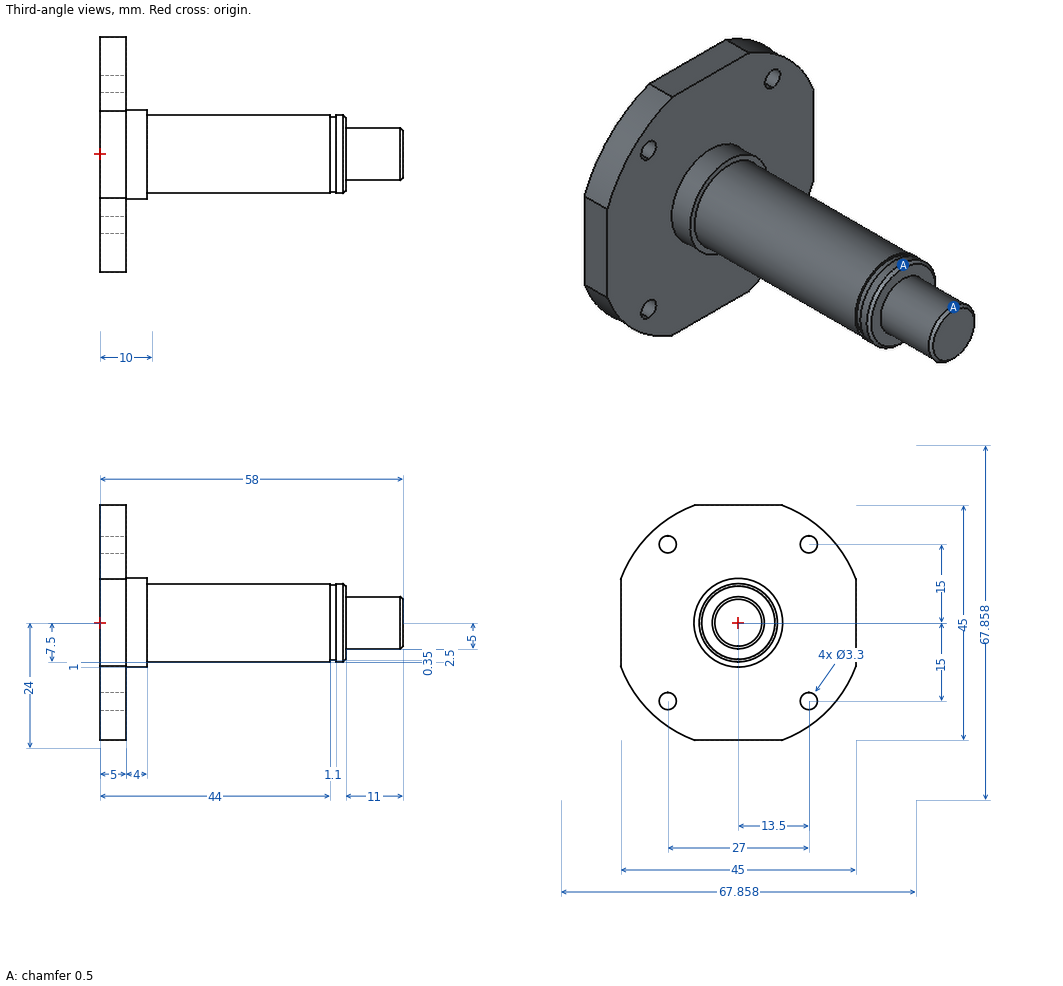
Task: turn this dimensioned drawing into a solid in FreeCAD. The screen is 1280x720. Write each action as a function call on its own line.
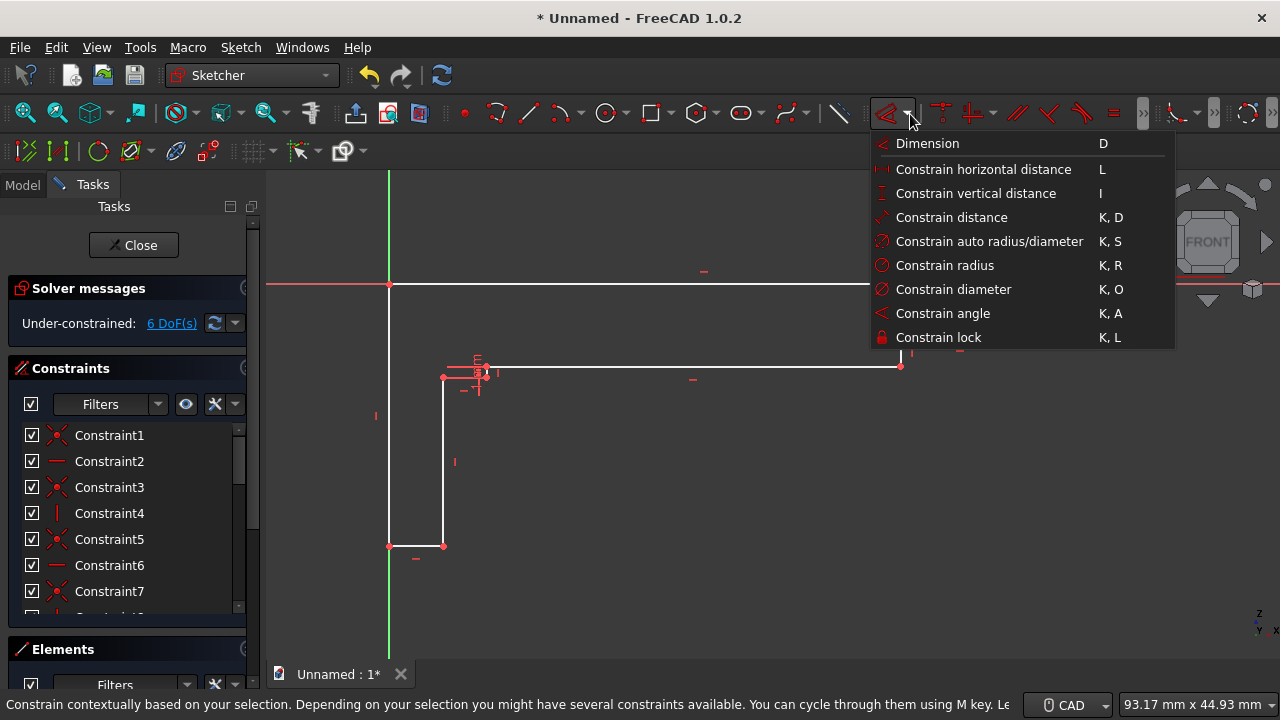
click(1023, 169)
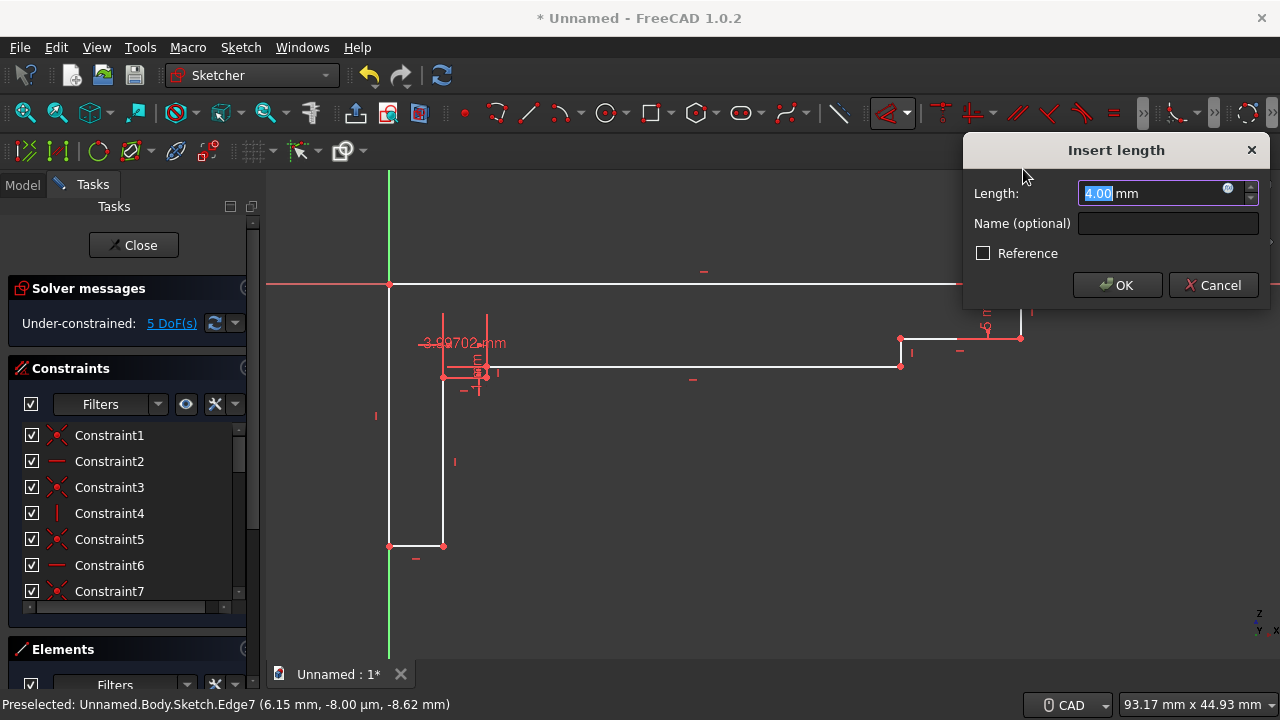
text(4)
key(Return)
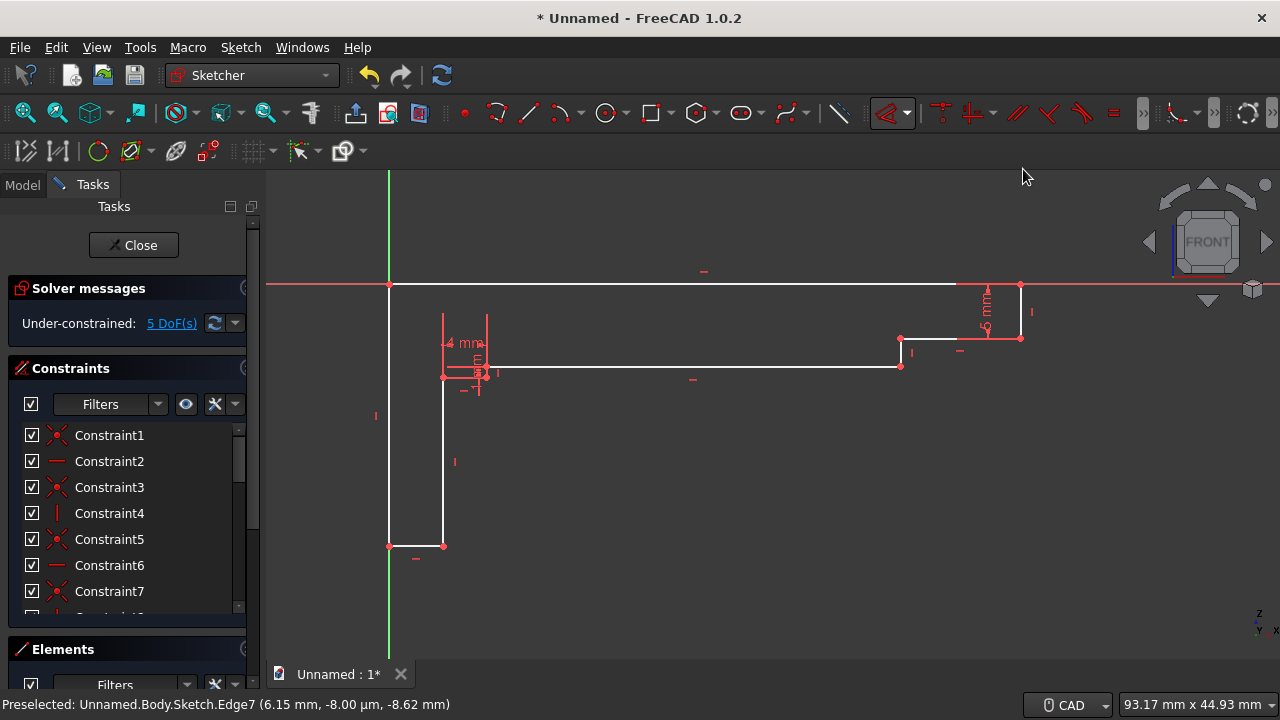
click(427, 546)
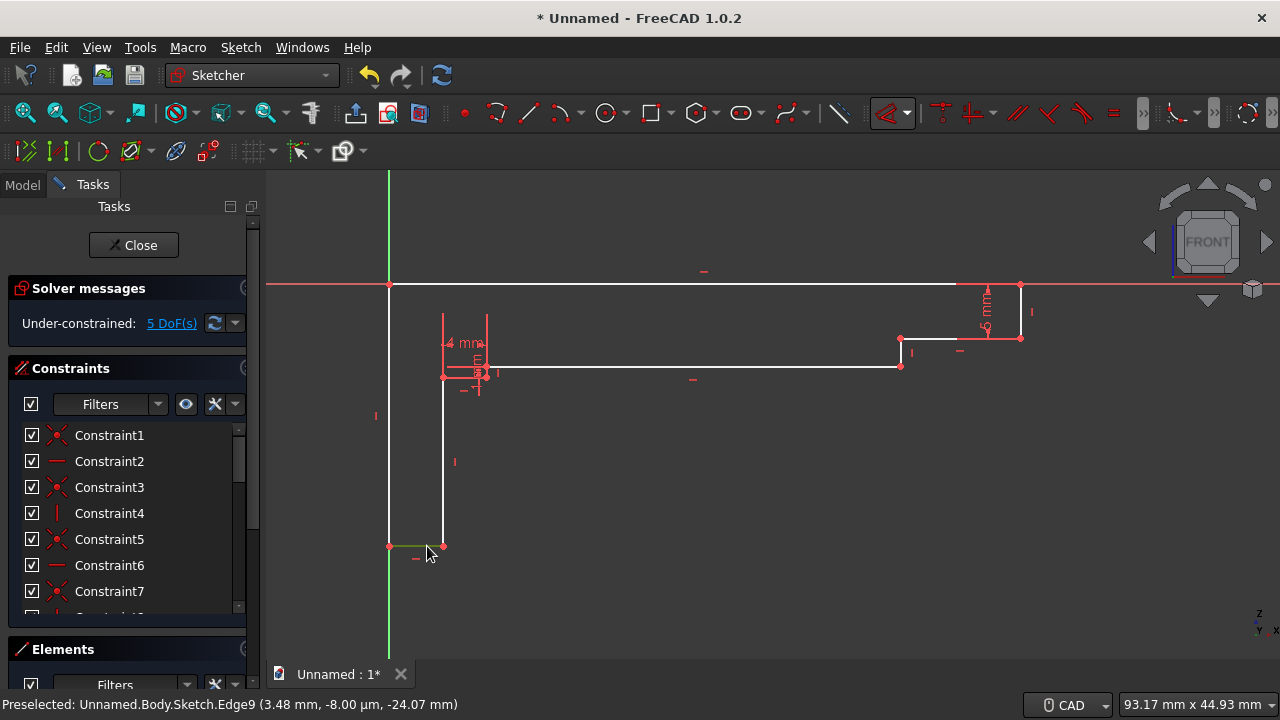
key(l)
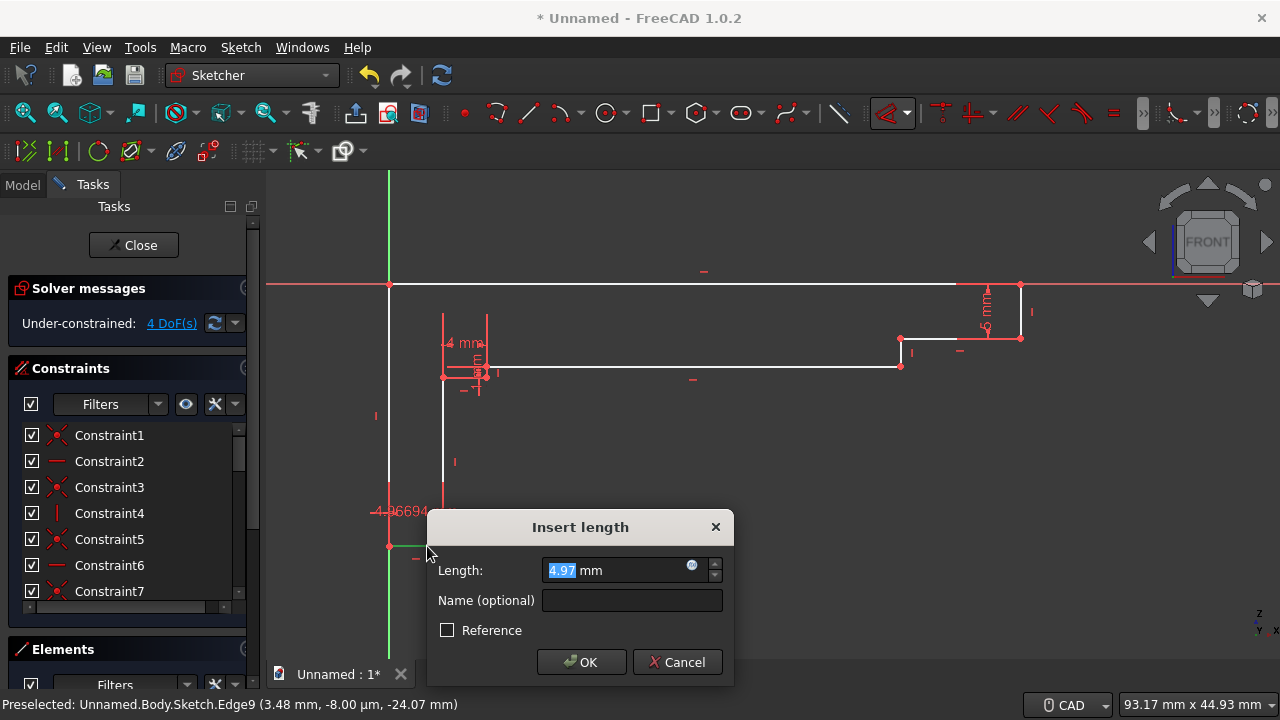
text(5)
key(Return)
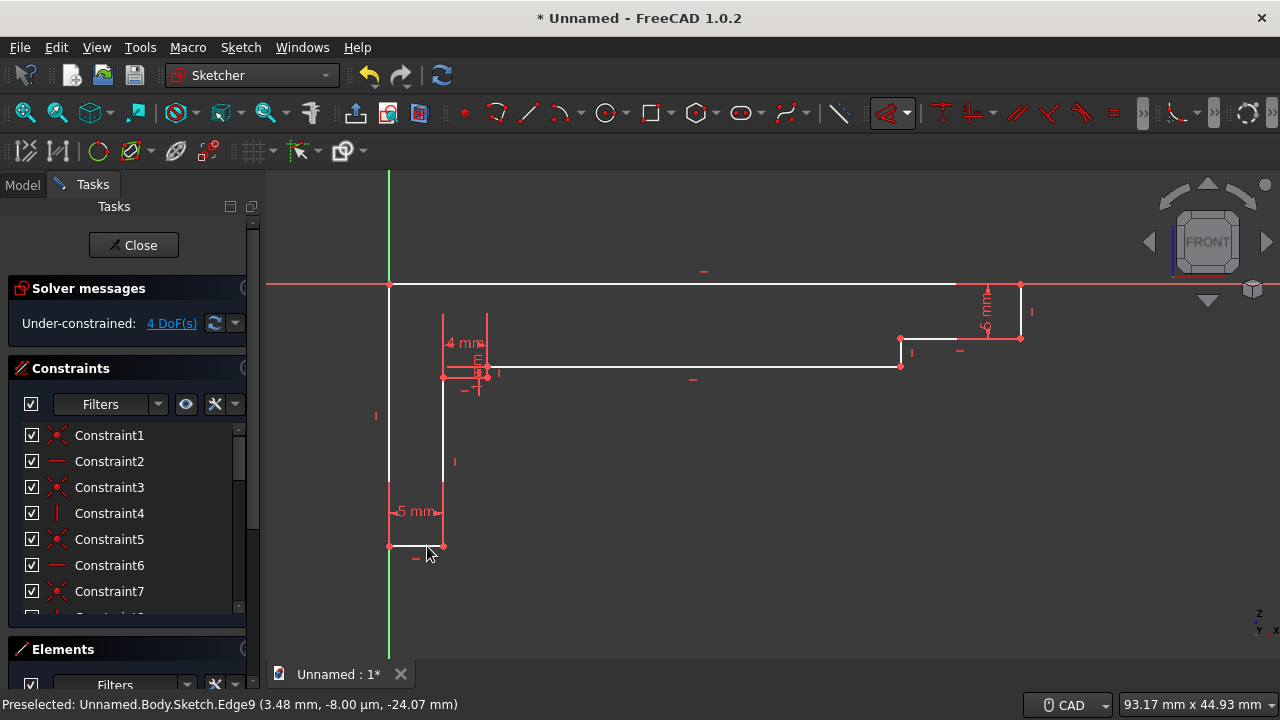
click(579, 284)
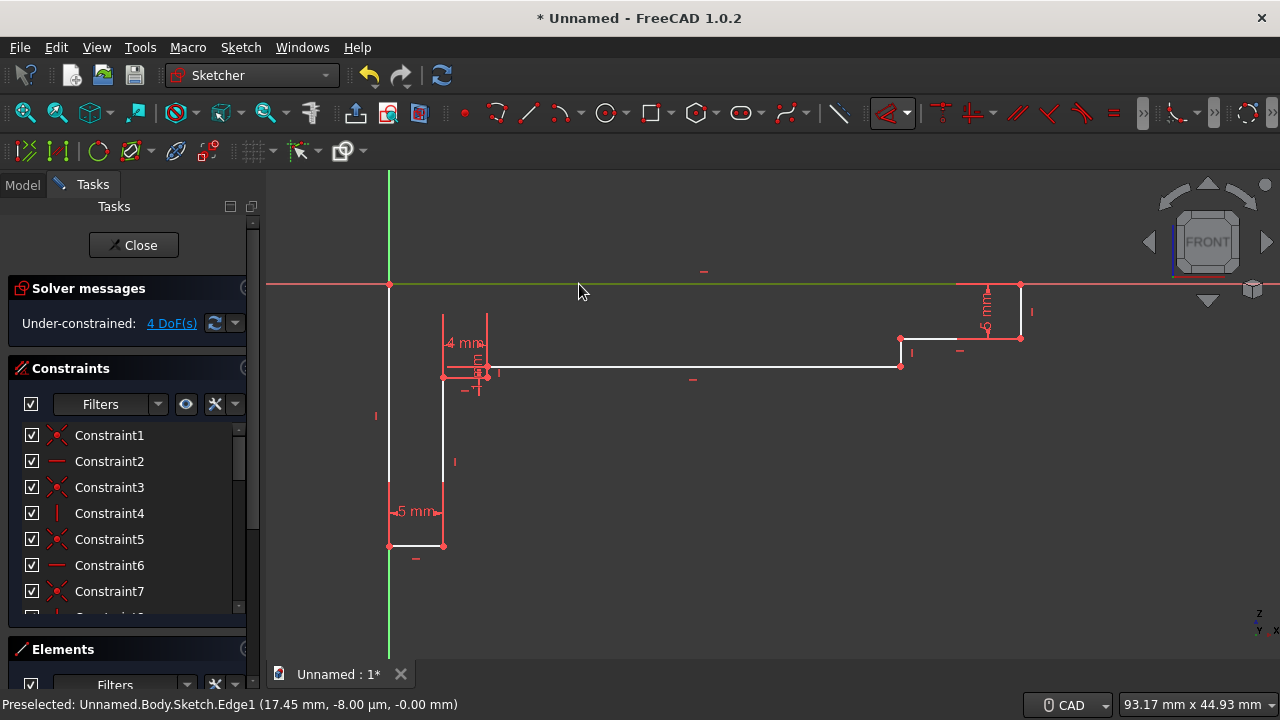
key(l)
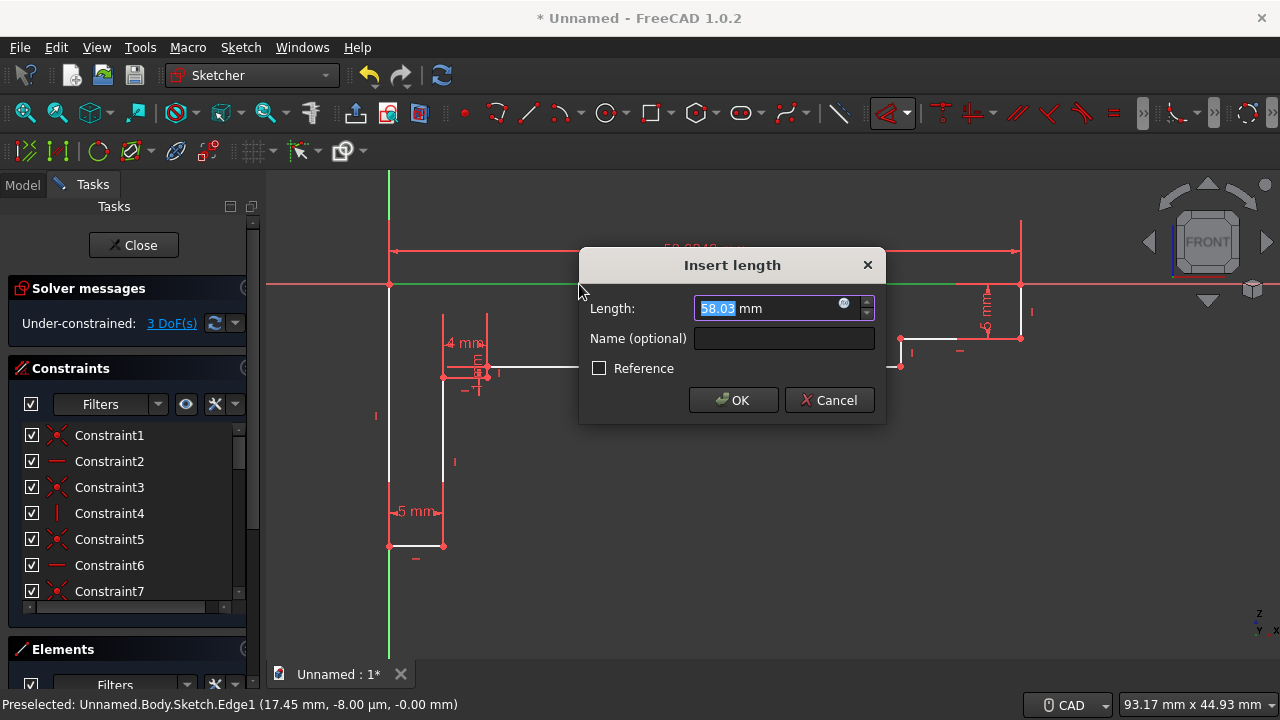
text(58)
key(Return)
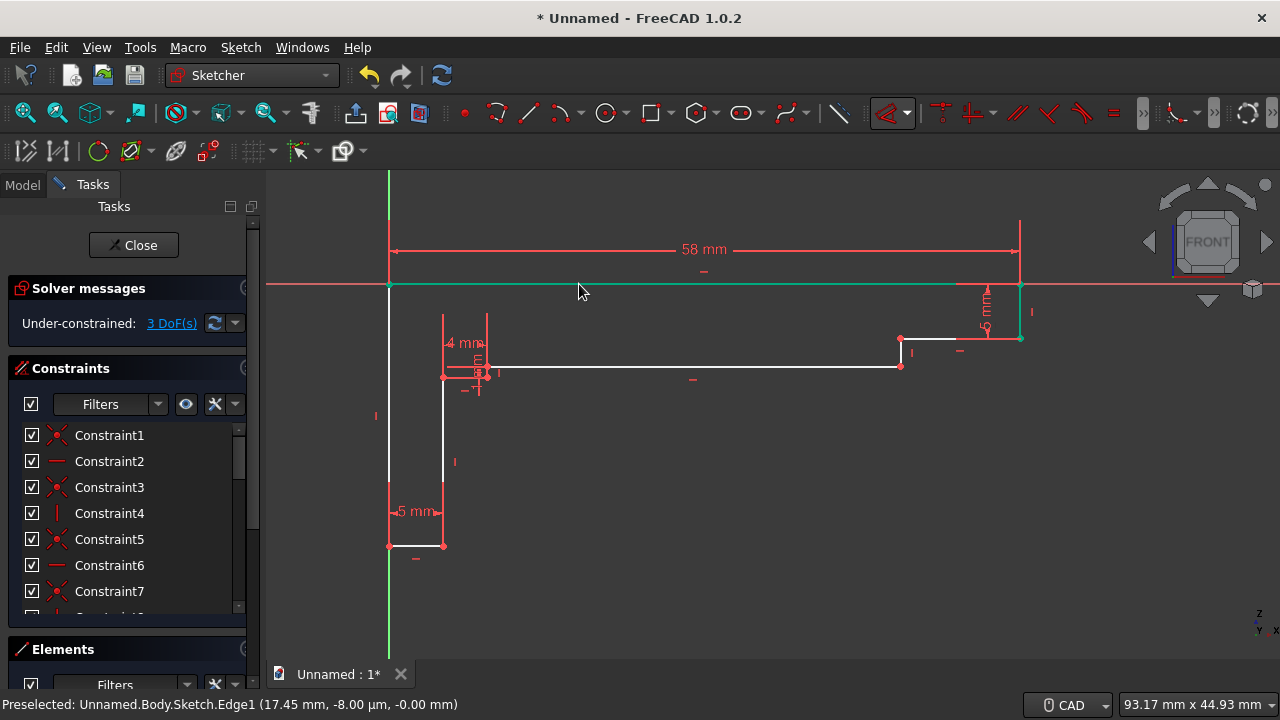
click(984, 339)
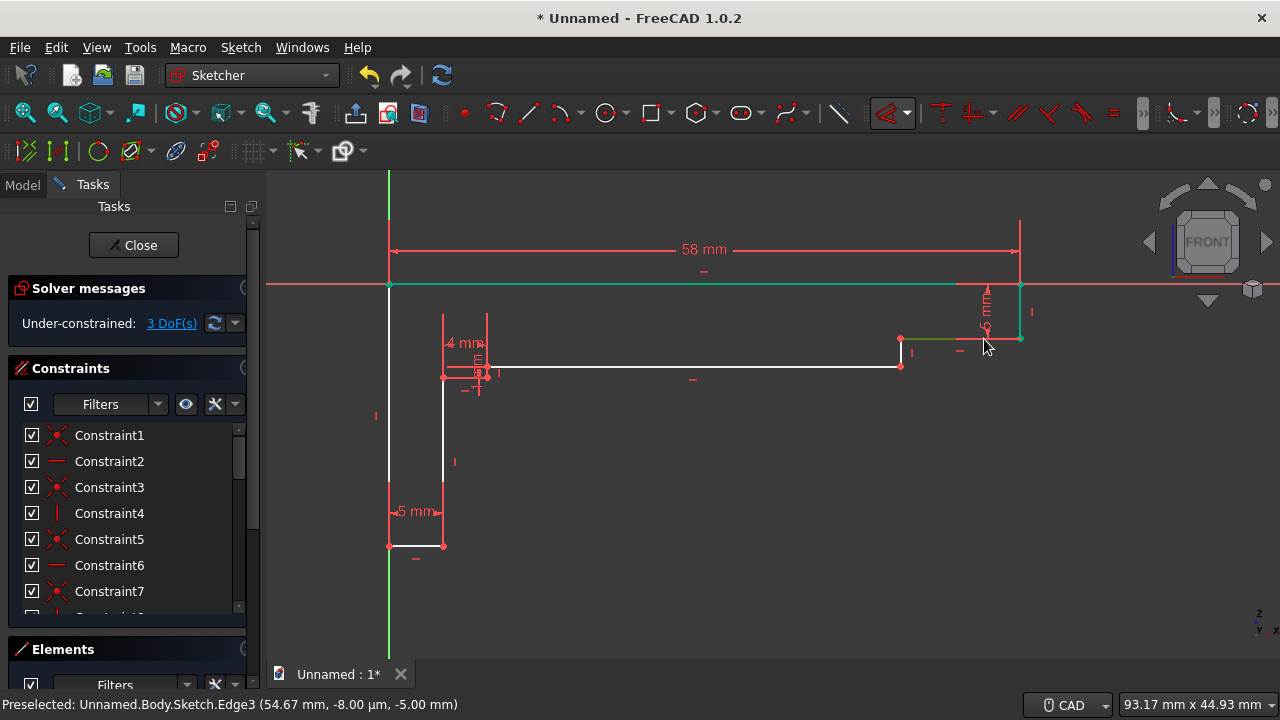
click(910, 114)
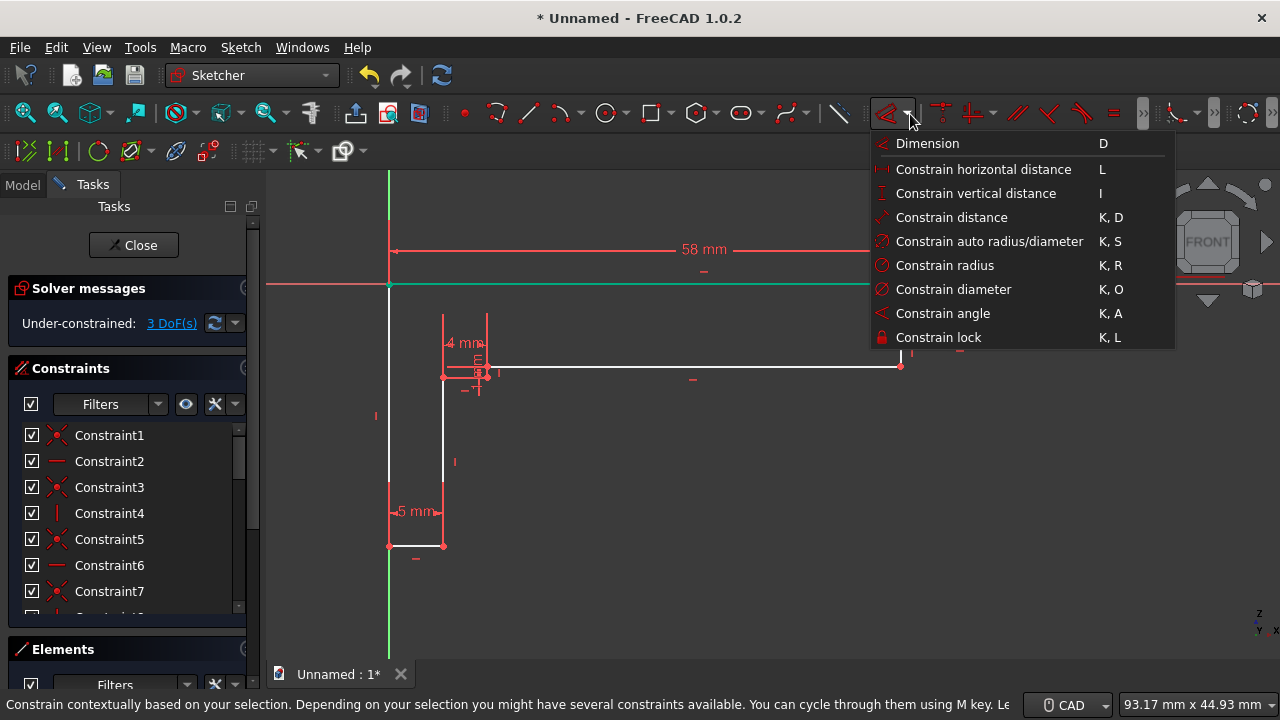
click(1023, 169)